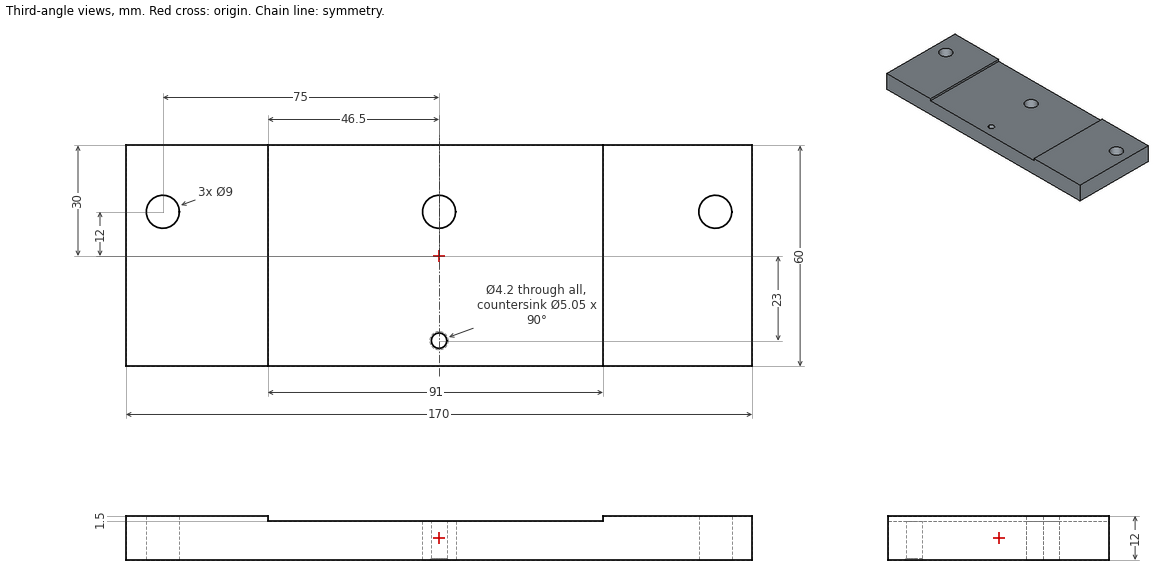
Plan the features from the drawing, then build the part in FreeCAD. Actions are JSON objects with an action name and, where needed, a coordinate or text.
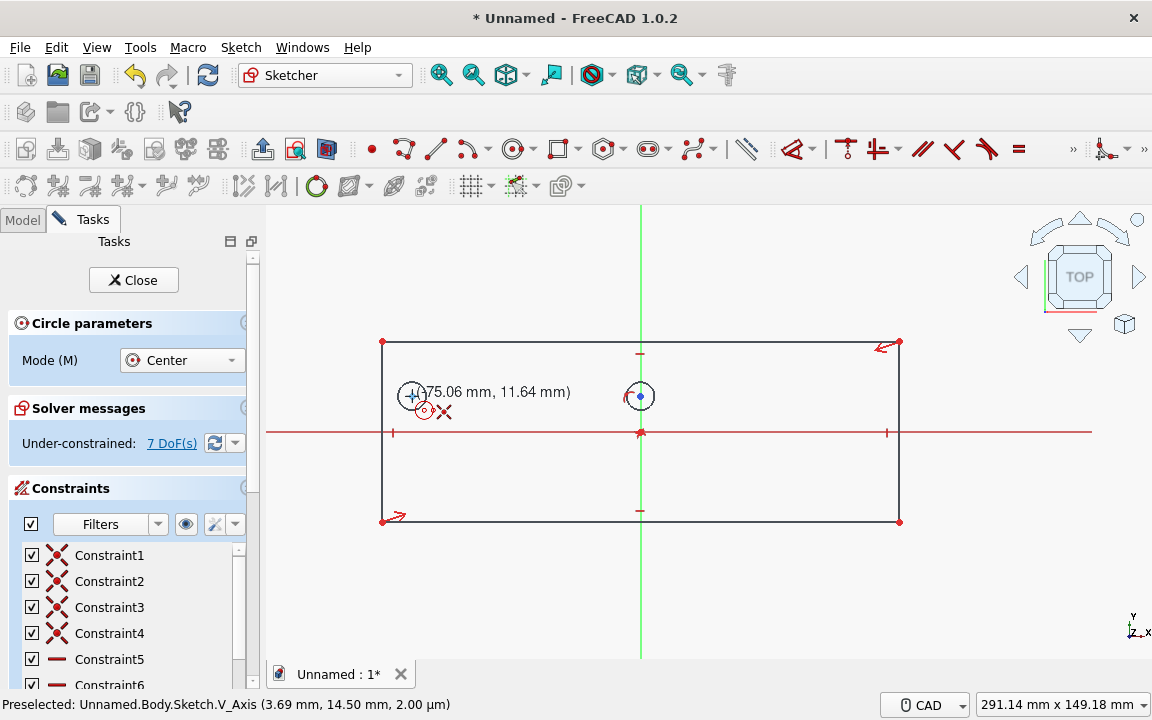
{"action": "scroll", "coordinate": [869, 396], "scroll_direction": "up", "scroll_amount": 3}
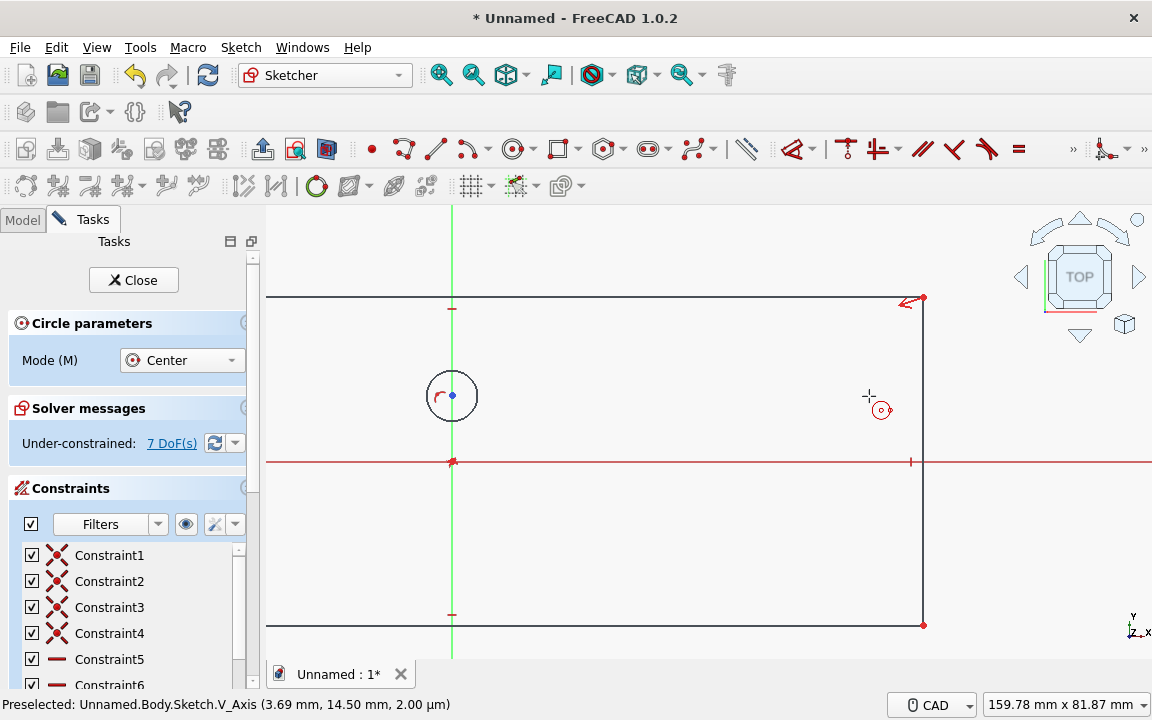
{"action": "left_click", "coordinate": [868, 395]}
{"action": "left_click", "coordinate": [886, 377]}
{"action": "key", "text": "Escape"}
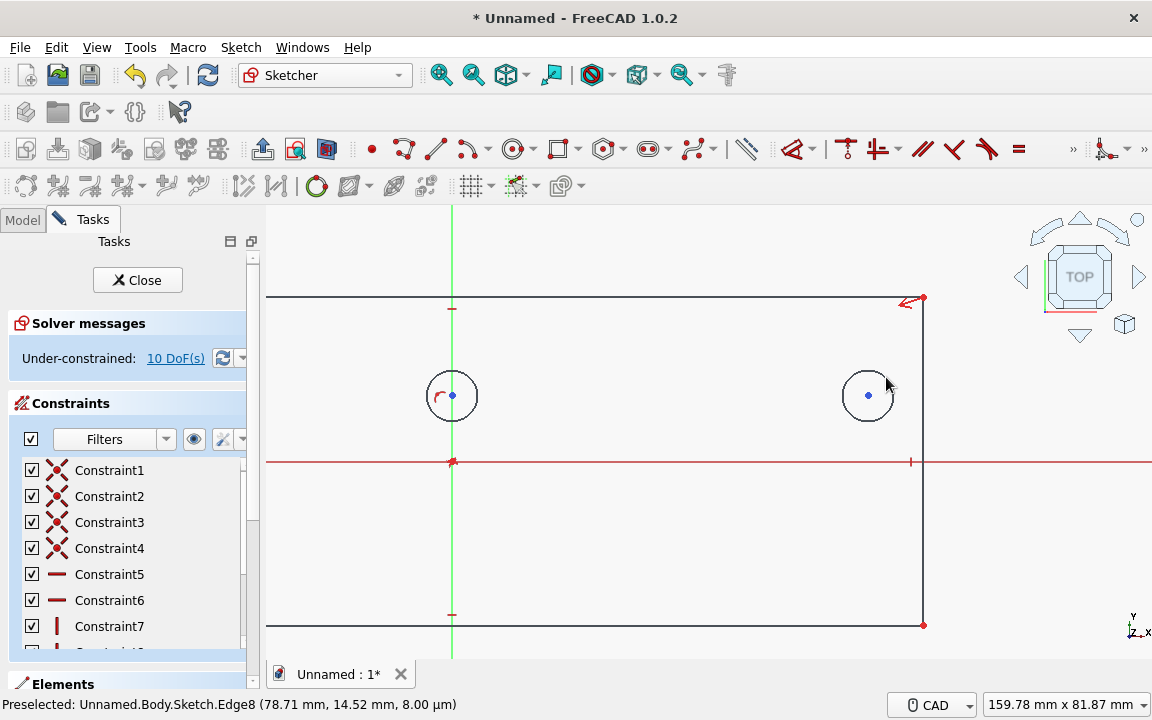
{"action": "scroll", "coordinate": [870, 396], "scroll_direction": "down", "scroll_amount": 3}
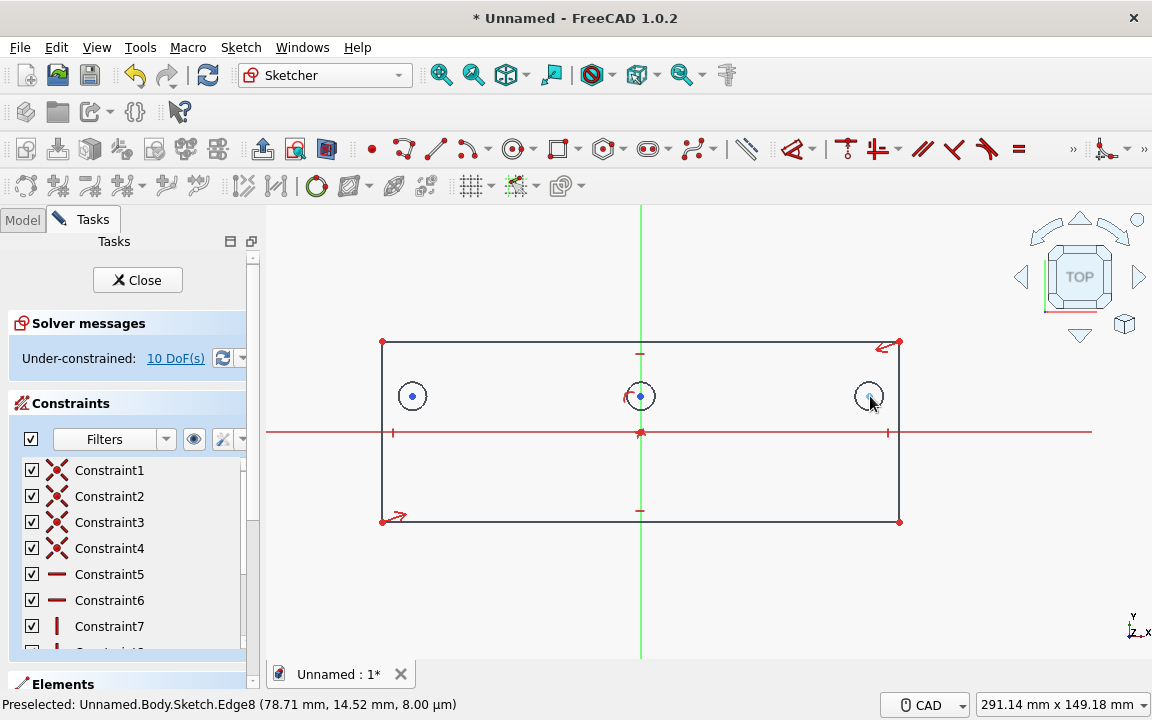
{"action": "left_click", "coordinate": [422, 386]}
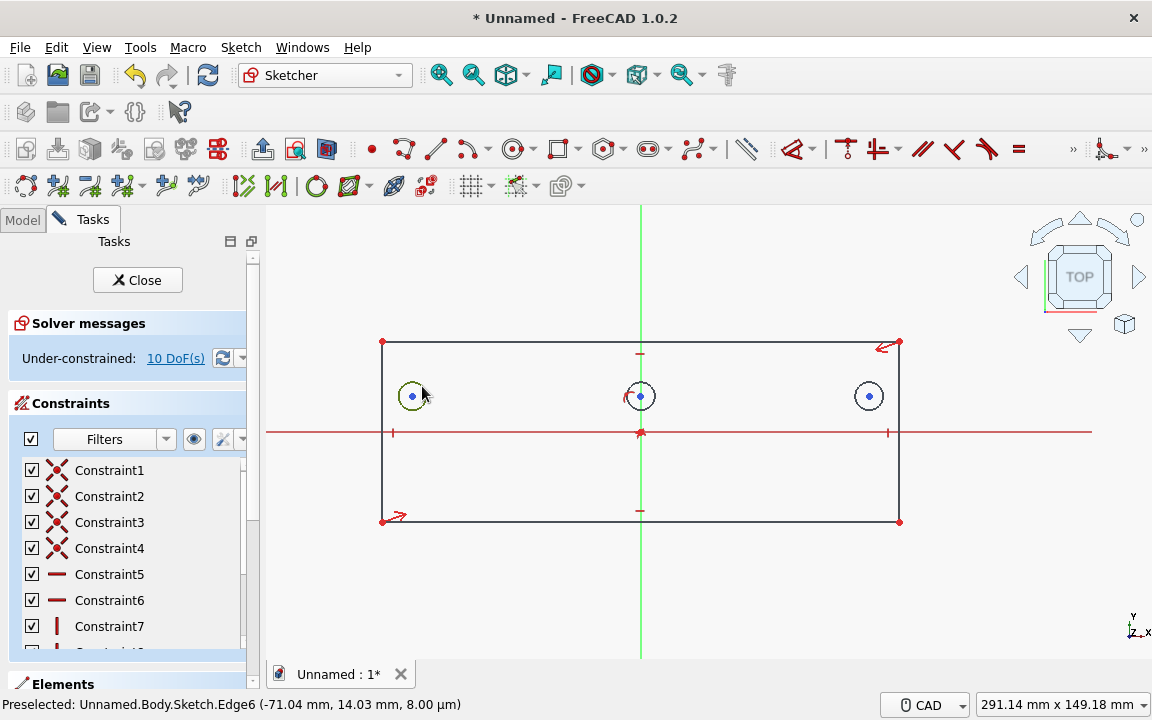
{"action": "scroll", "coordinate": [651, 386], "scroll_direction": "up", "scroll_amount": 2}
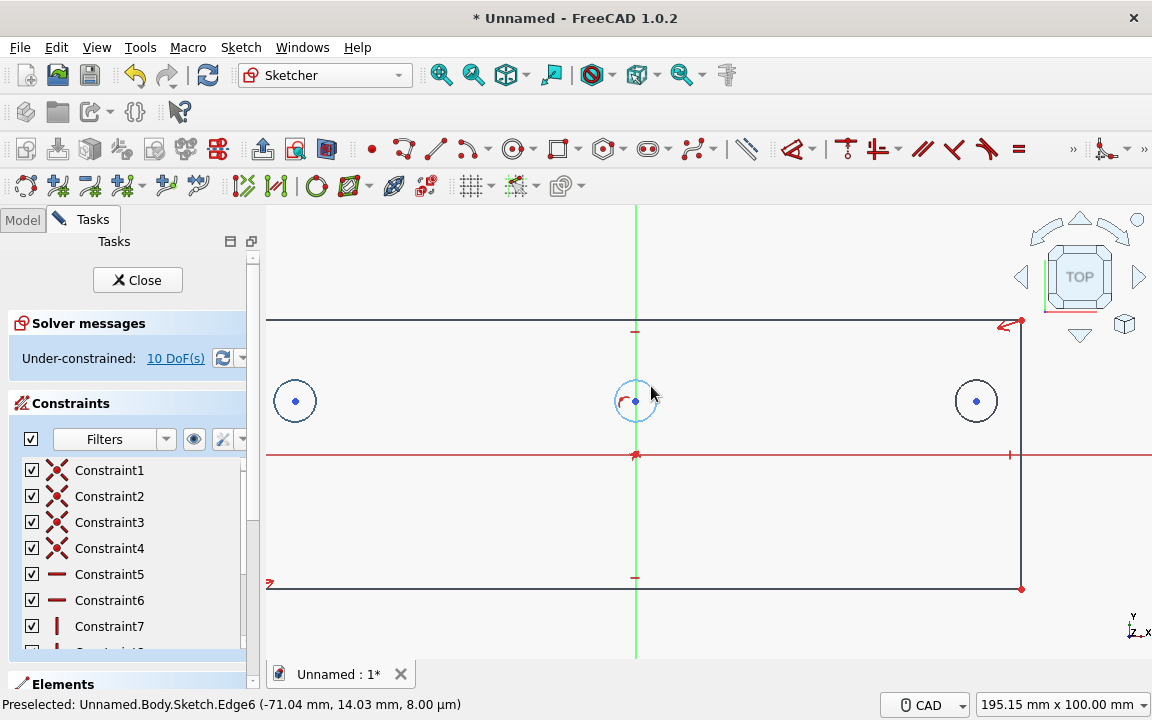
{"action": "left_click", "coordinate": [650, 386]}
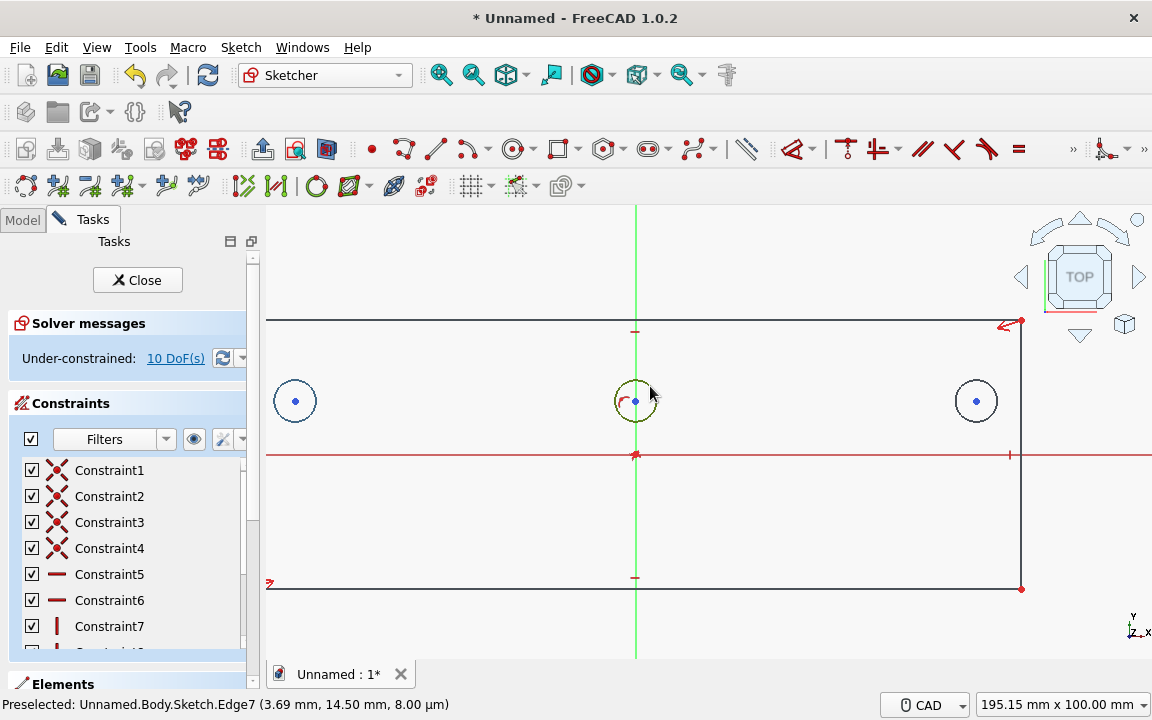
{"action": "left_click", "coordinate": [962, 386]}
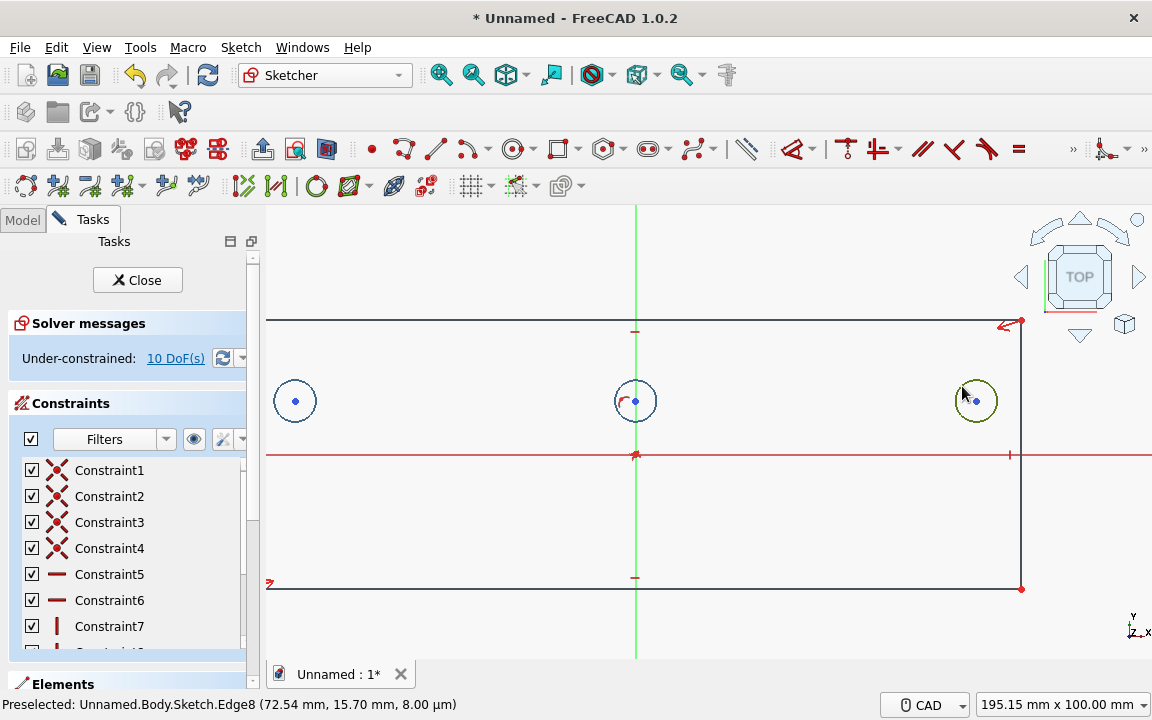
{"action": "key", "text": "e"}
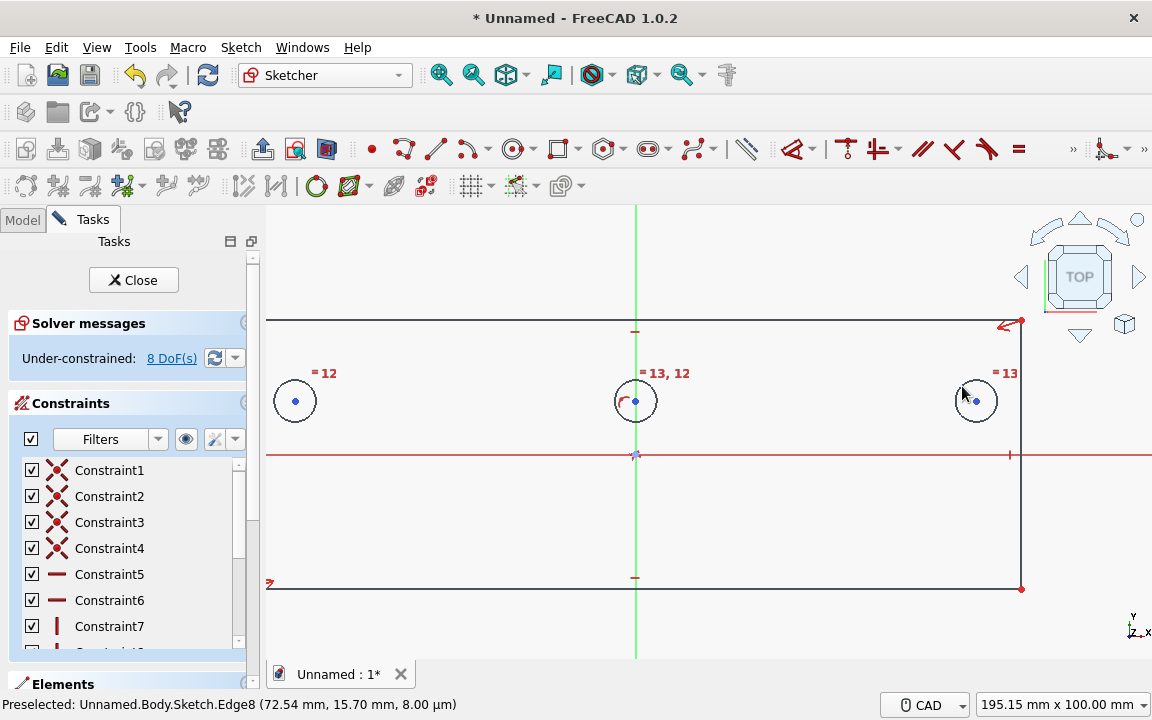
{"action": "left_click", "coordinate": [295, 401]}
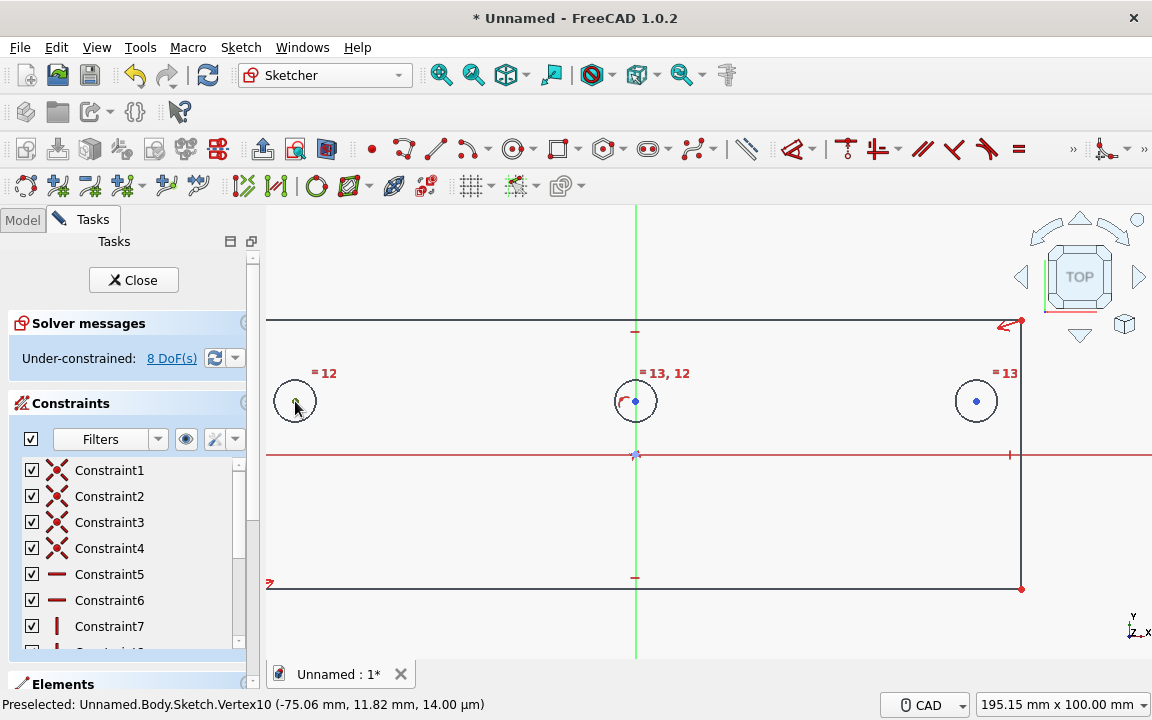
{"action": "left_click", "coordinate": [976, 401]}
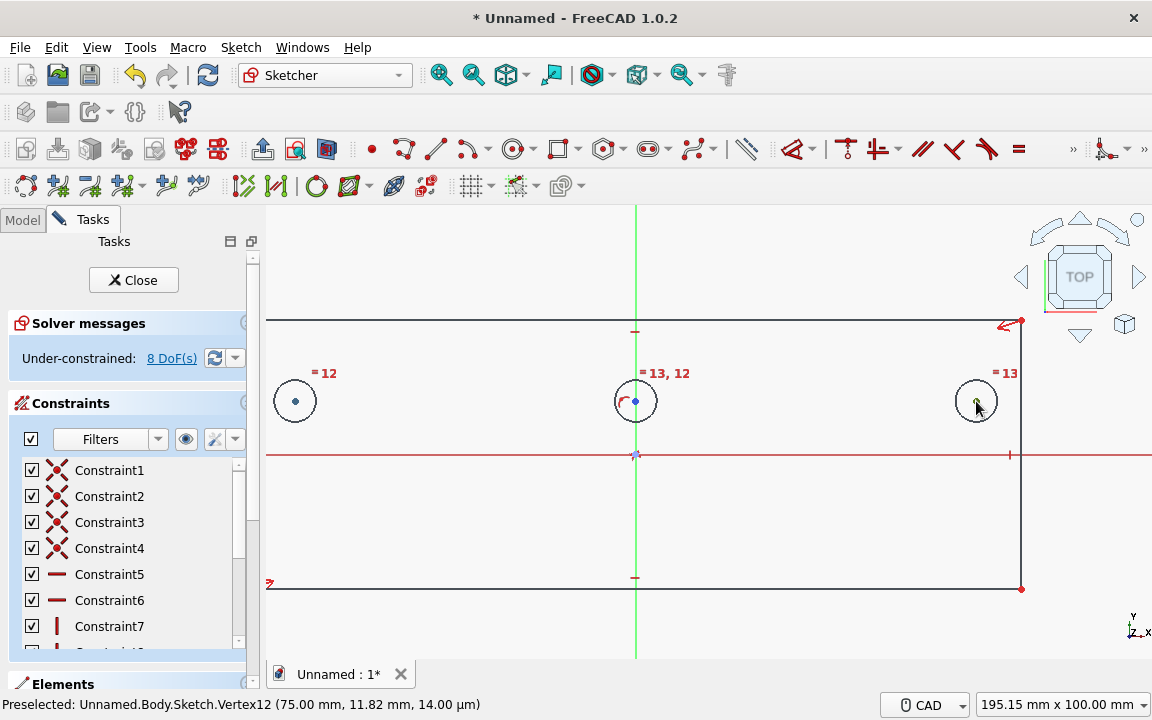
{"action": "left_click", "coordinate": [636, 546]}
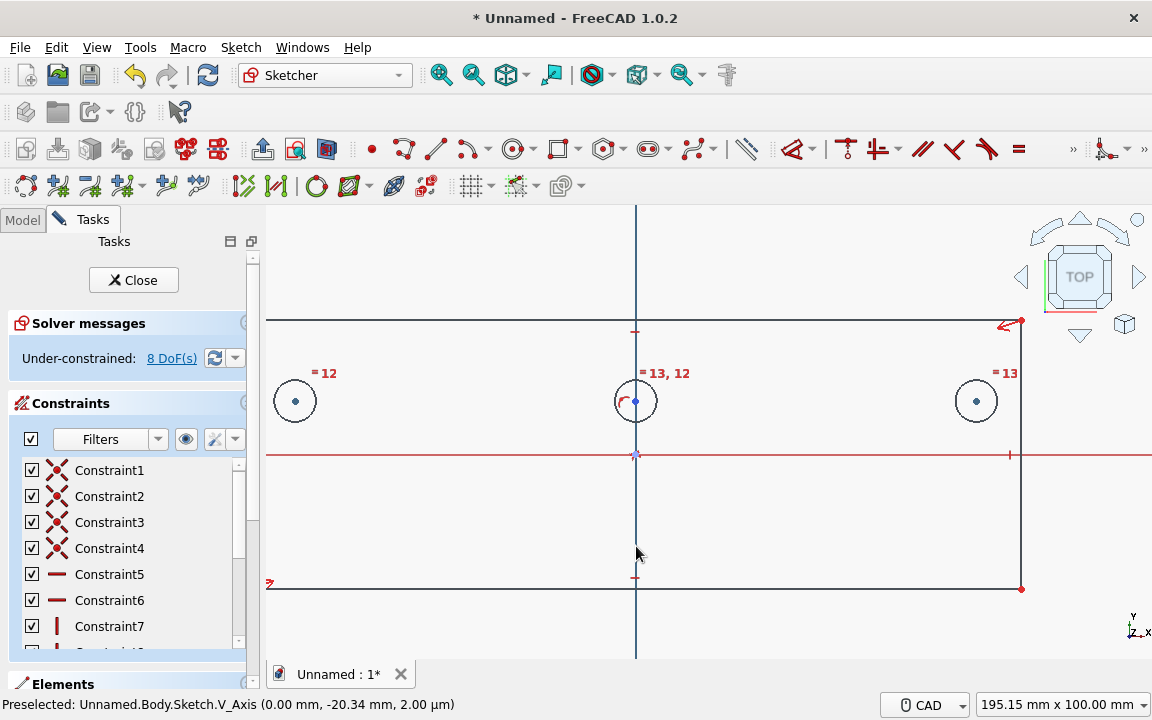
{"action": "key", "text": "s"}